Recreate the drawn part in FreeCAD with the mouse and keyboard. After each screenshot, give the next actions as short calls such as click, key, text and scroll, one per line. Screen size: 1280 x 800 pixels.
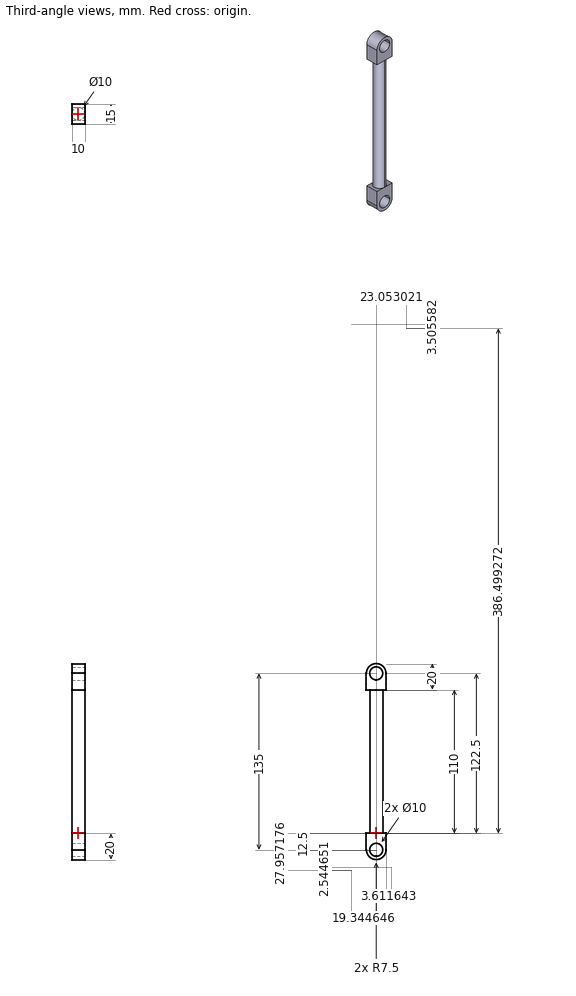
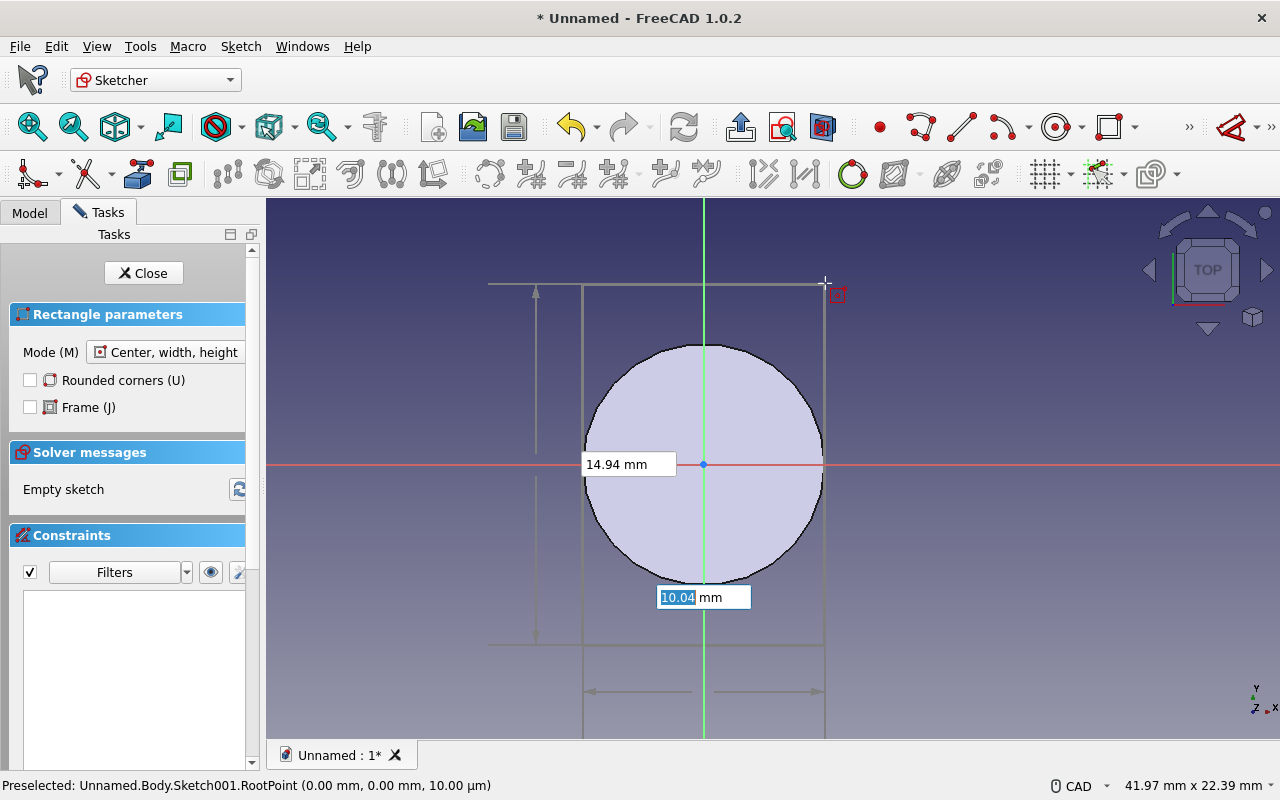
text(10)
key(Tab)
text(15)
key(Return)
key(Escape)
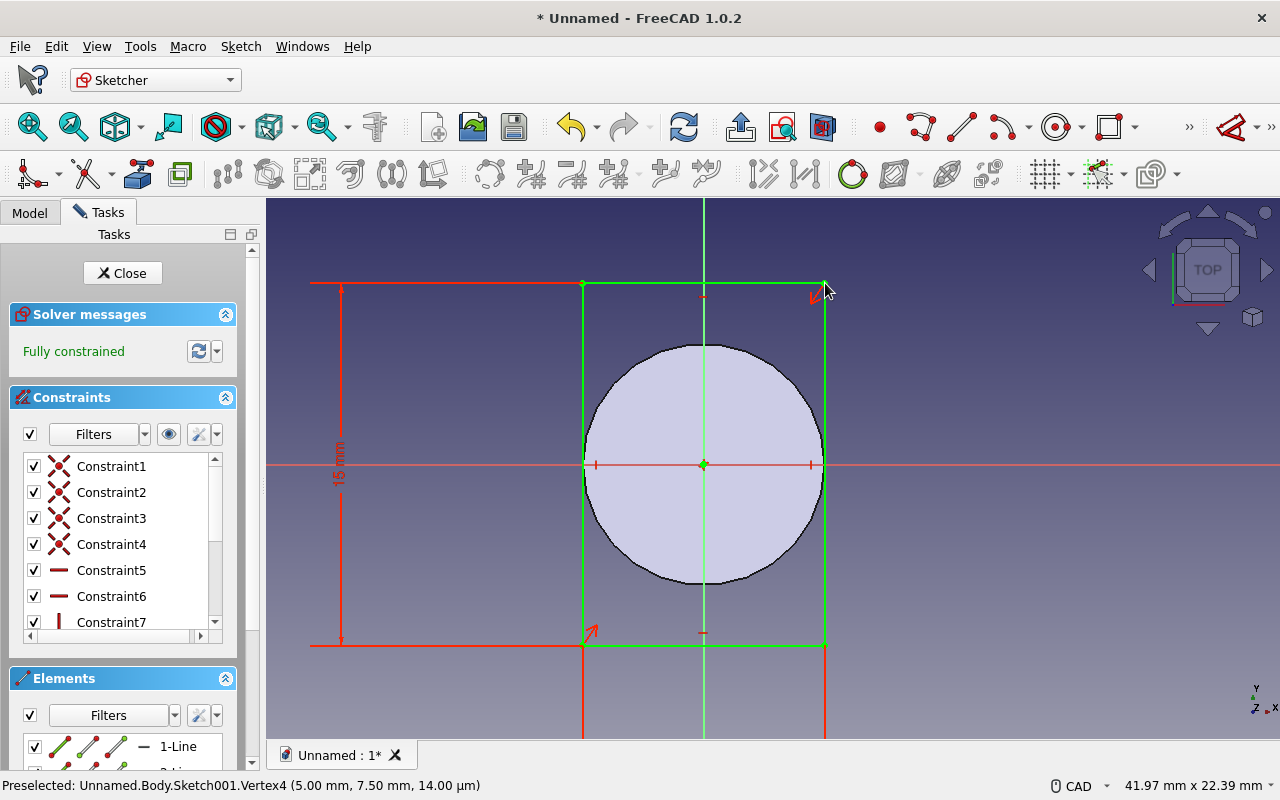
click(123, 273)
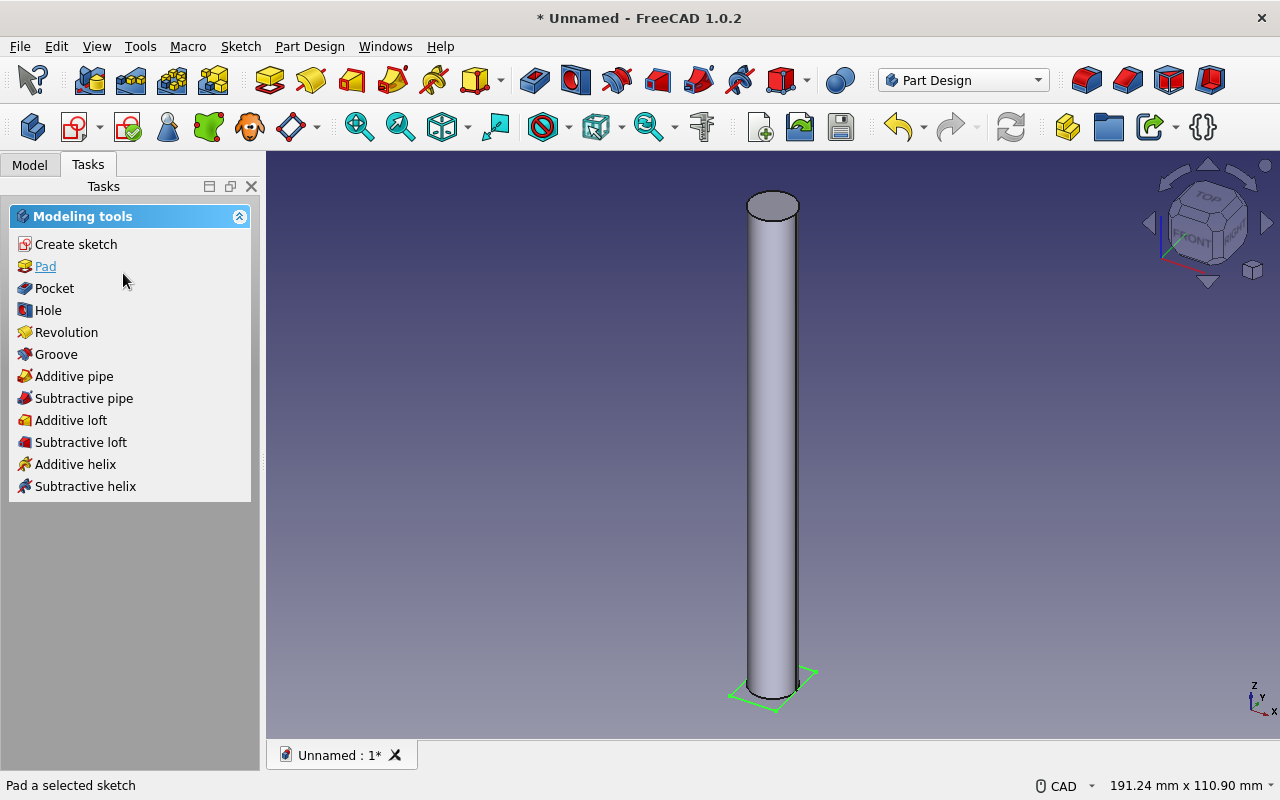
click(270, 80)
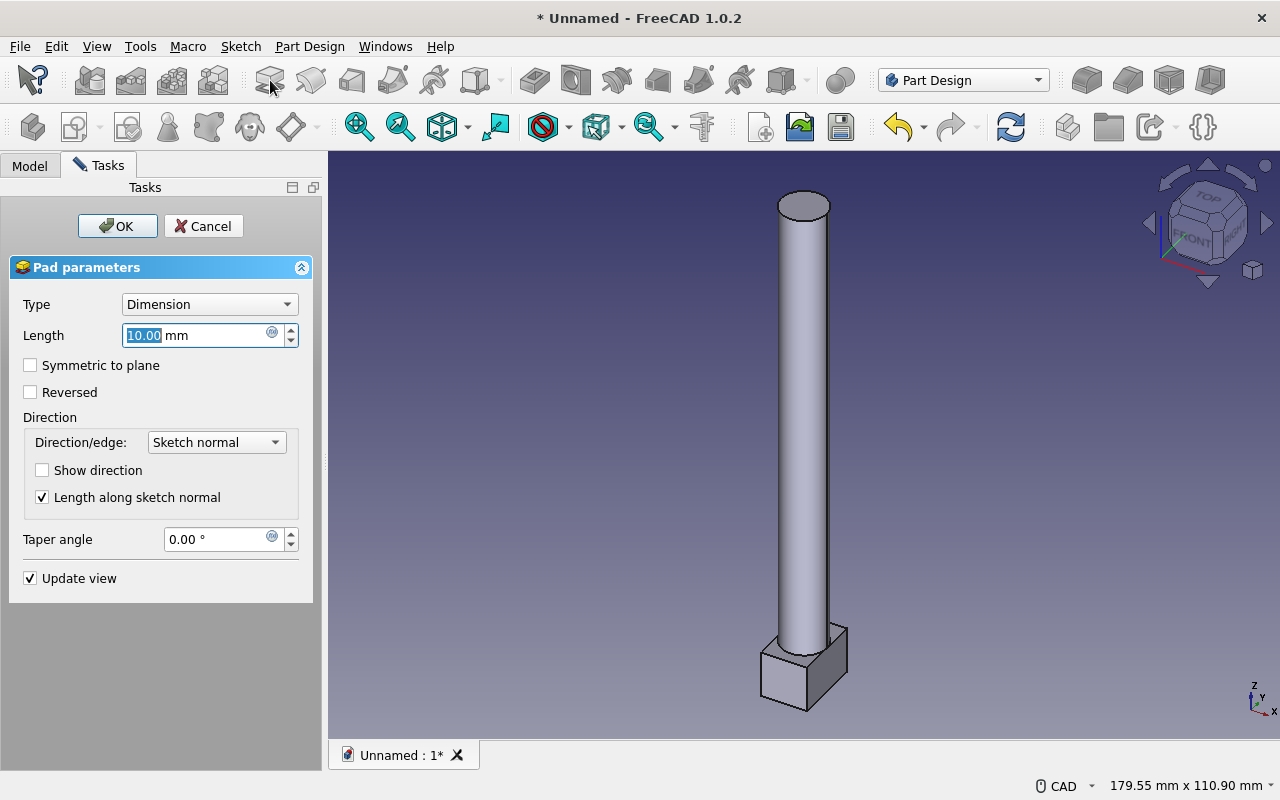
text(20)
key(Tab)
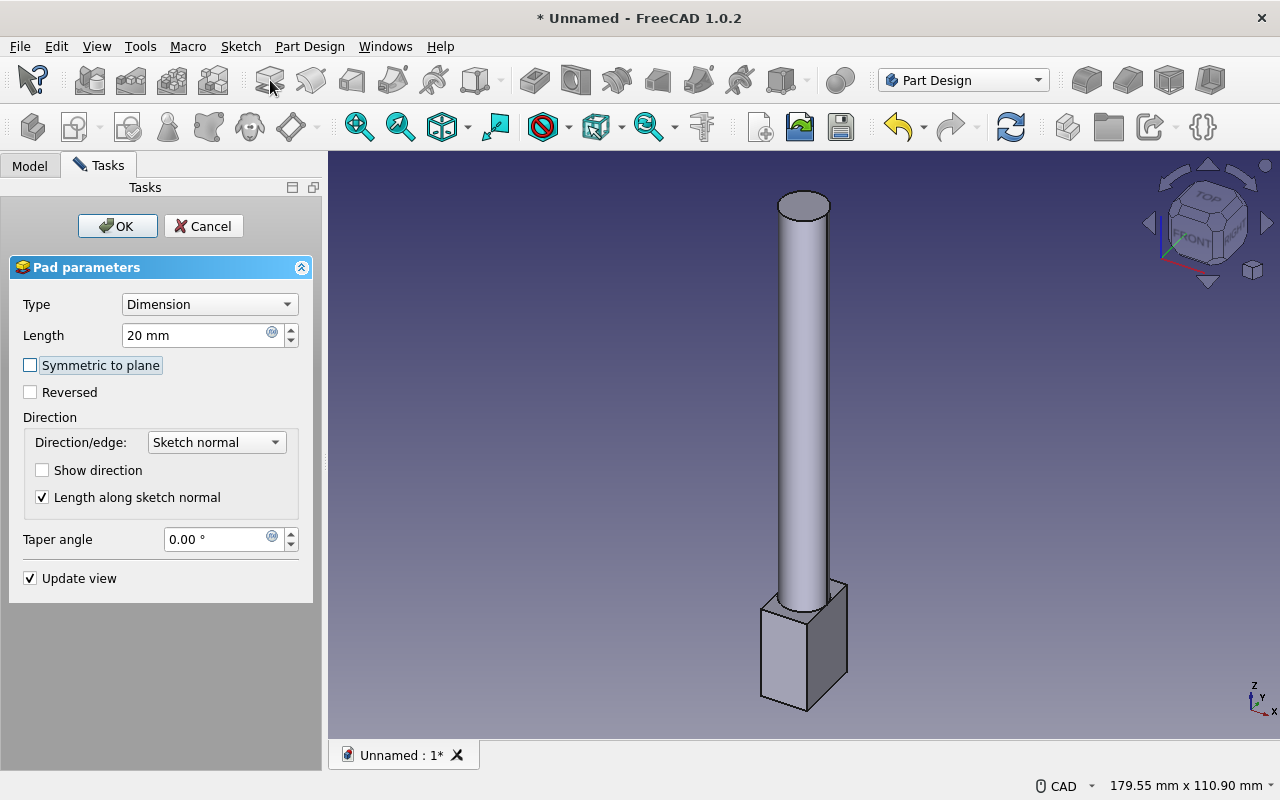
click(31, 392)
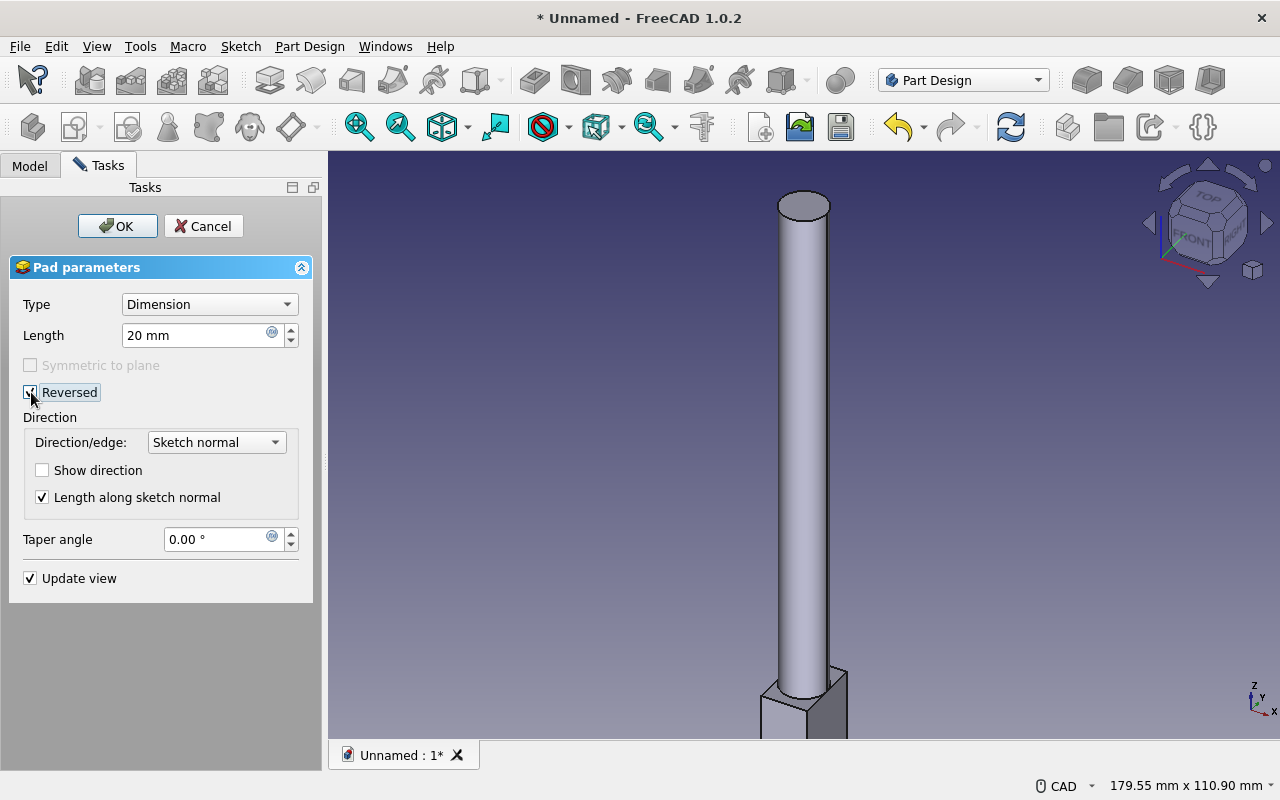
click(118, 226)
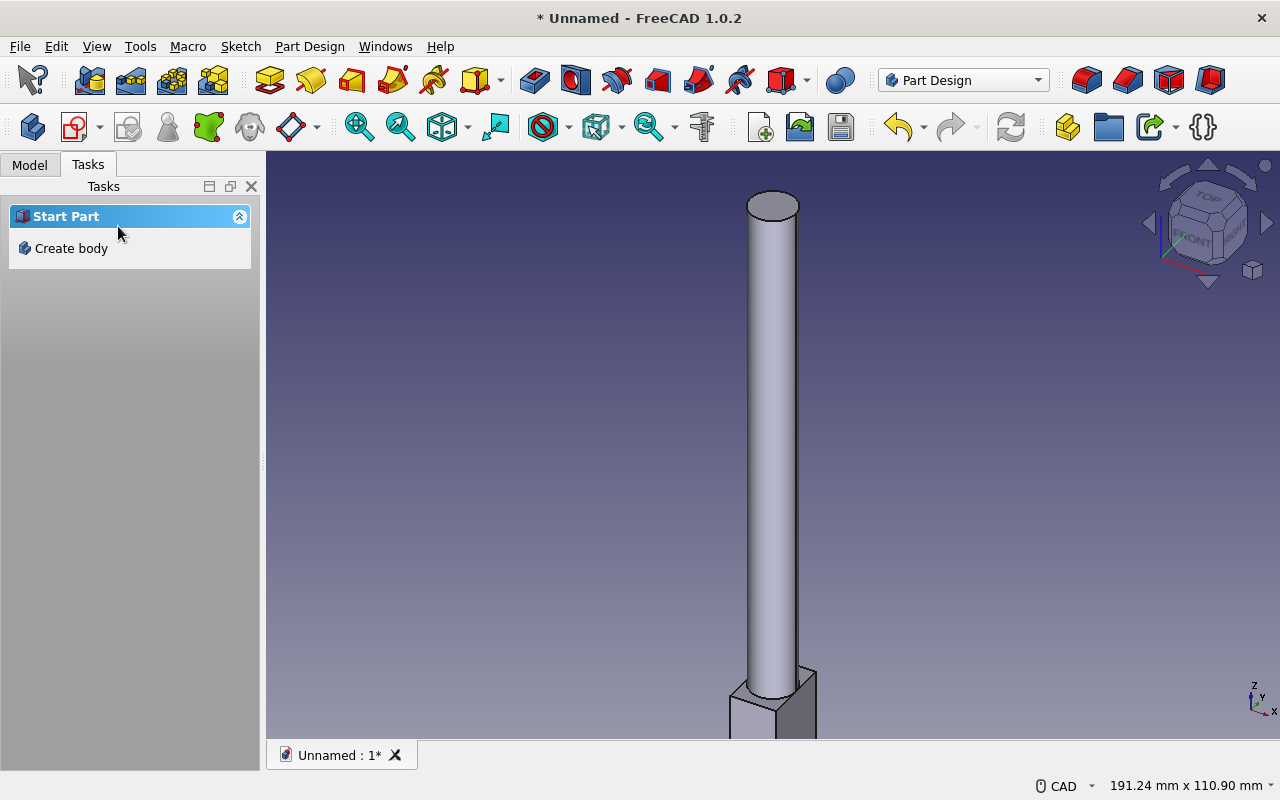
click(360, 128)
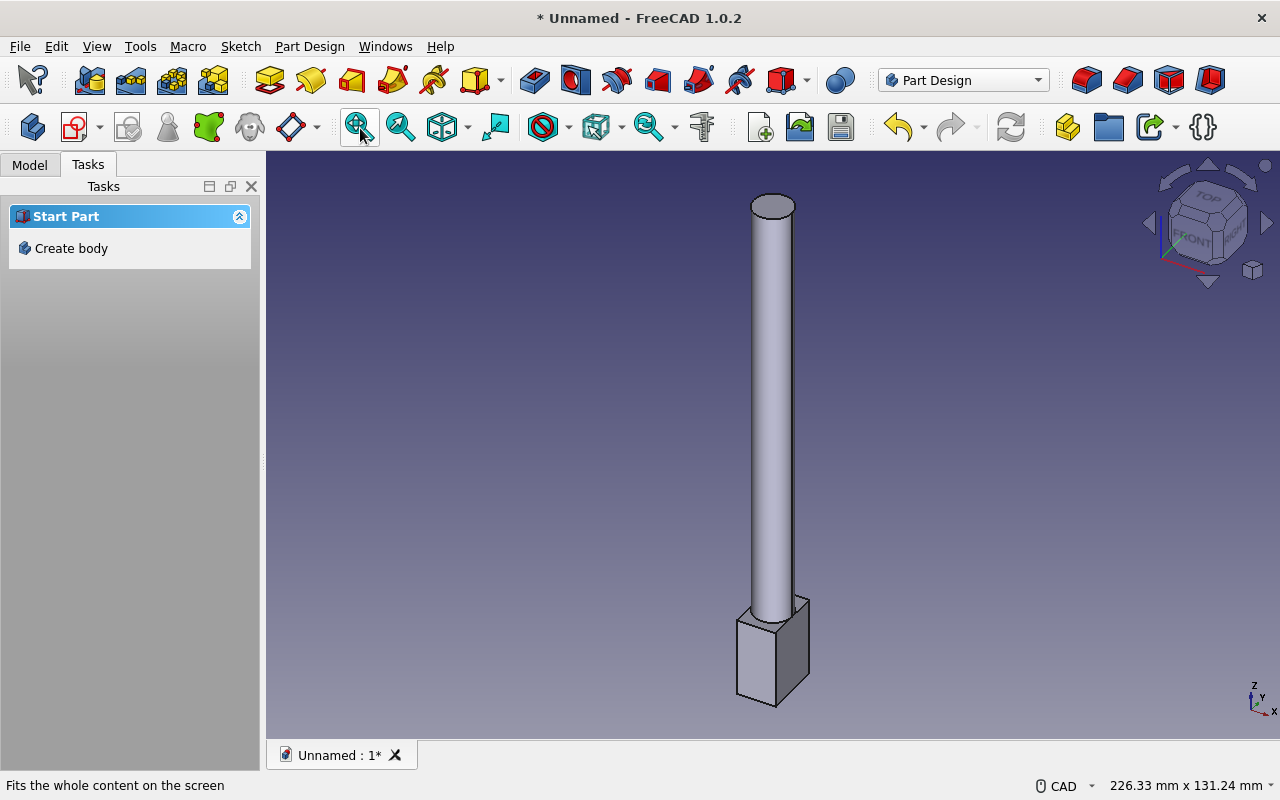
click(773, 205)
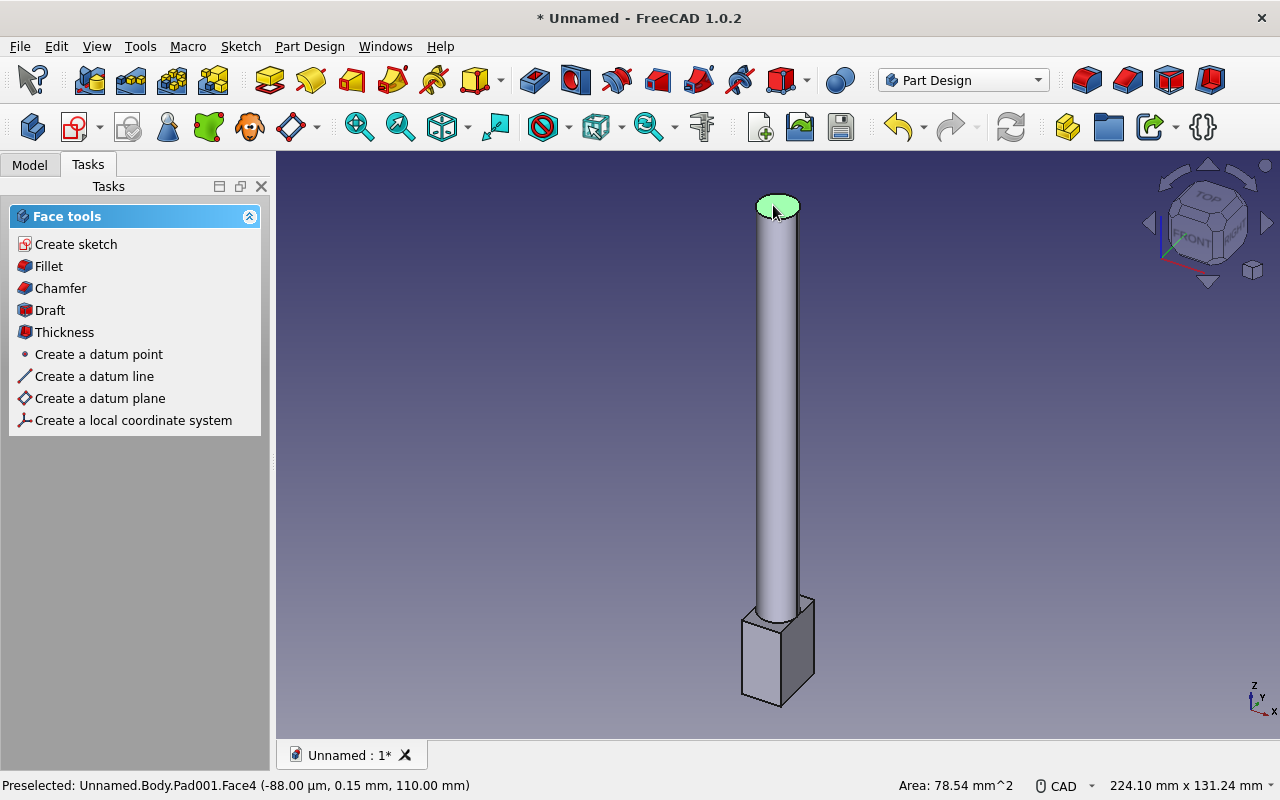
click(74, 128)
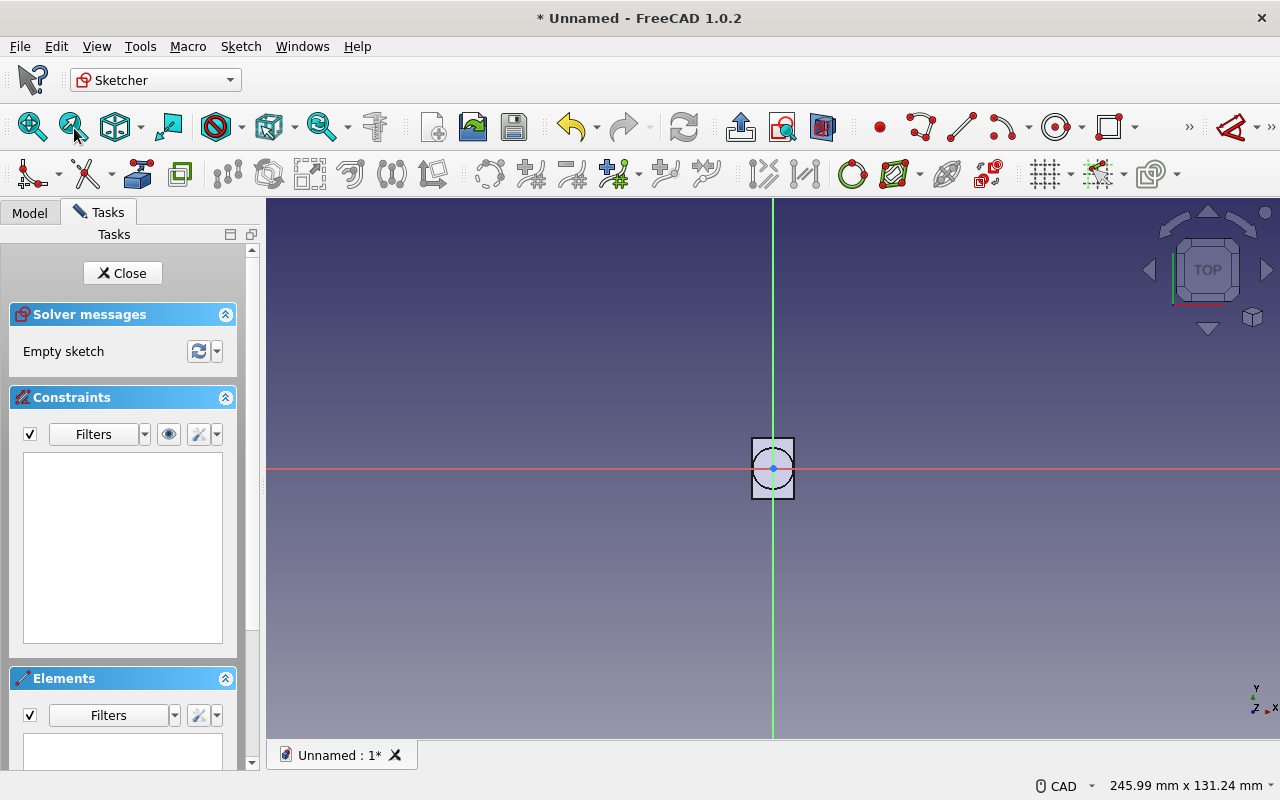
scroll(787, 468, up, 9)